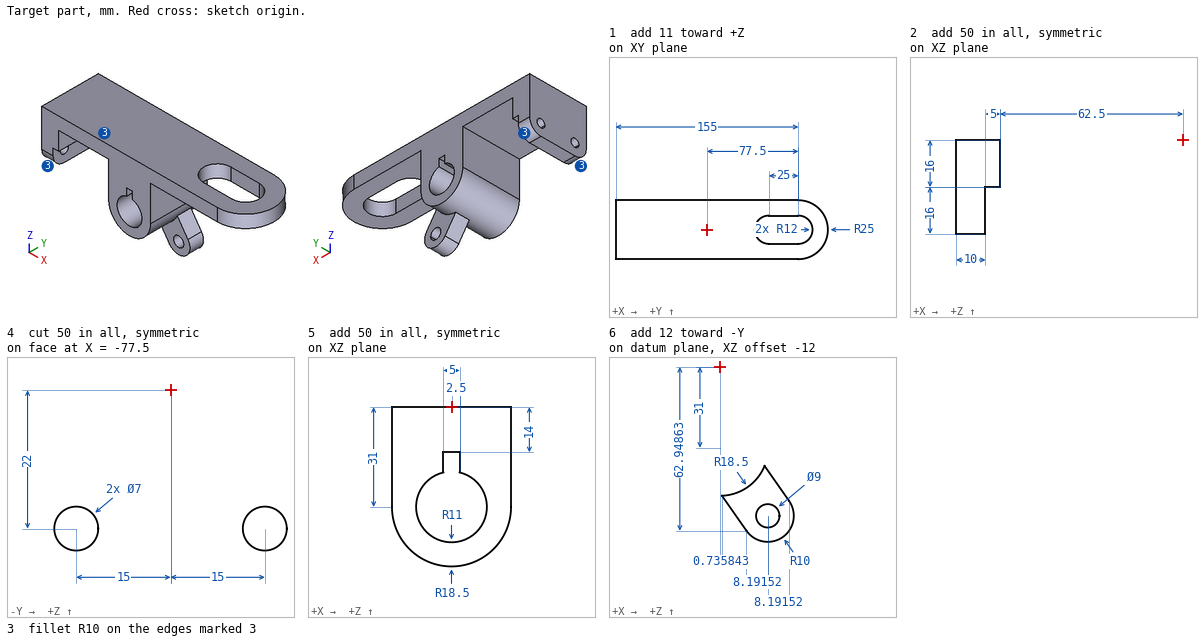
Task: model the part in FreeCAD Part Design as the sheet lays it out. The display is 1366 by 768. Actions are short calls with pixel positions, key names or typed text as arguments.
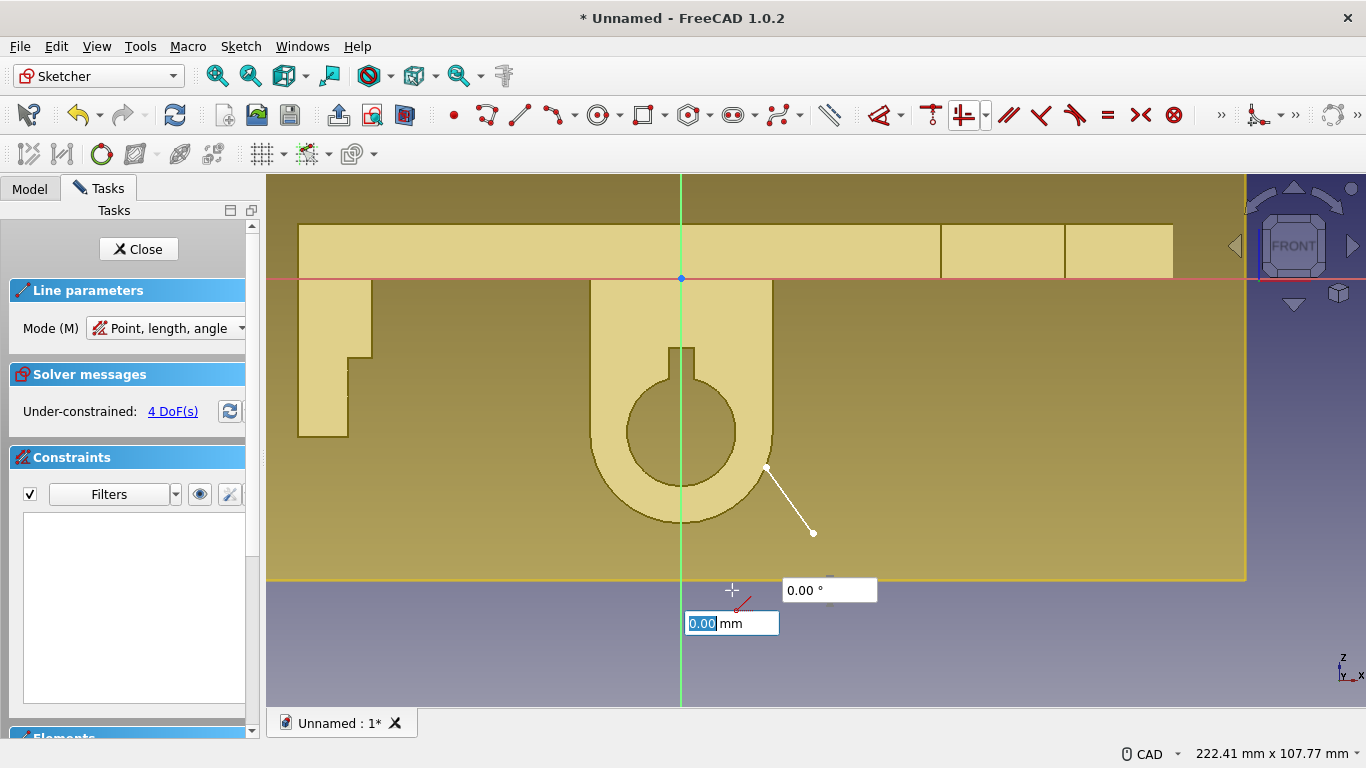
scroll(685, 523, up, 8)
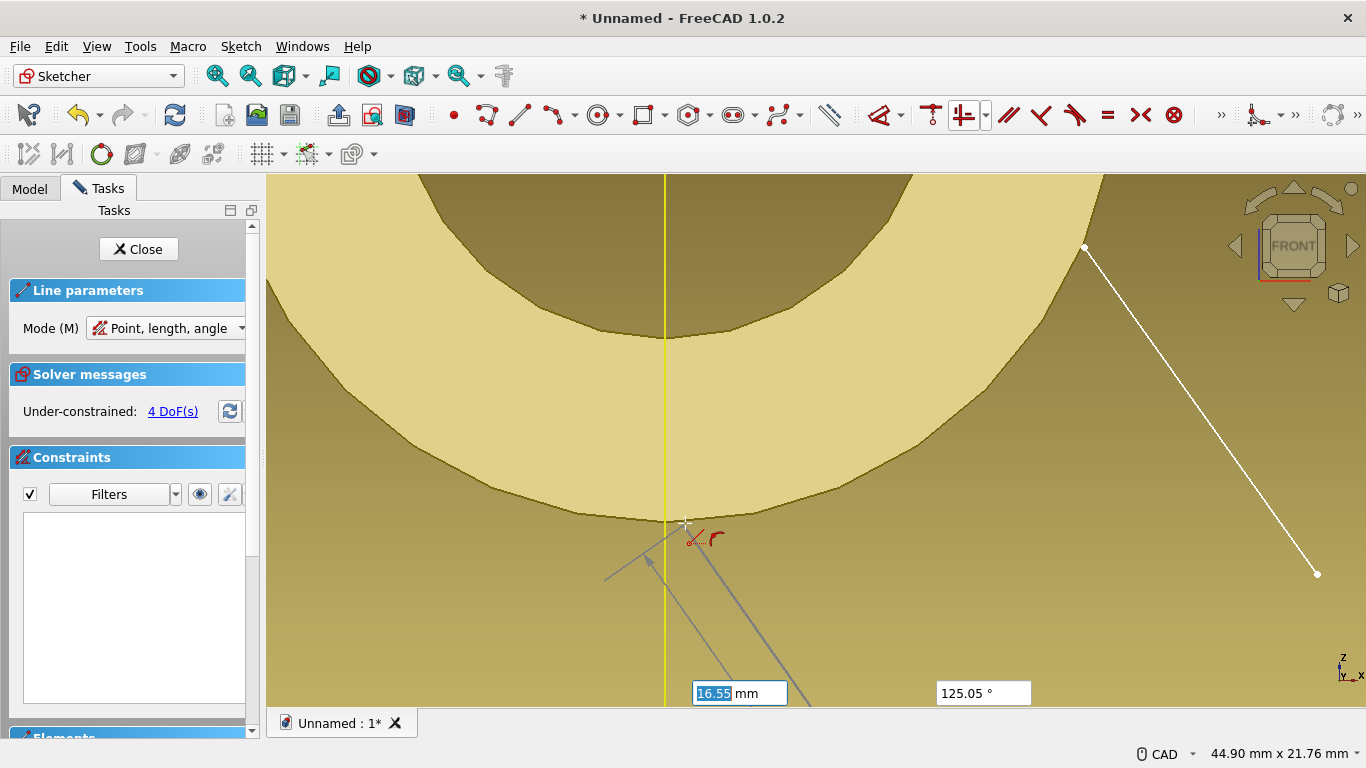
click(683, 522)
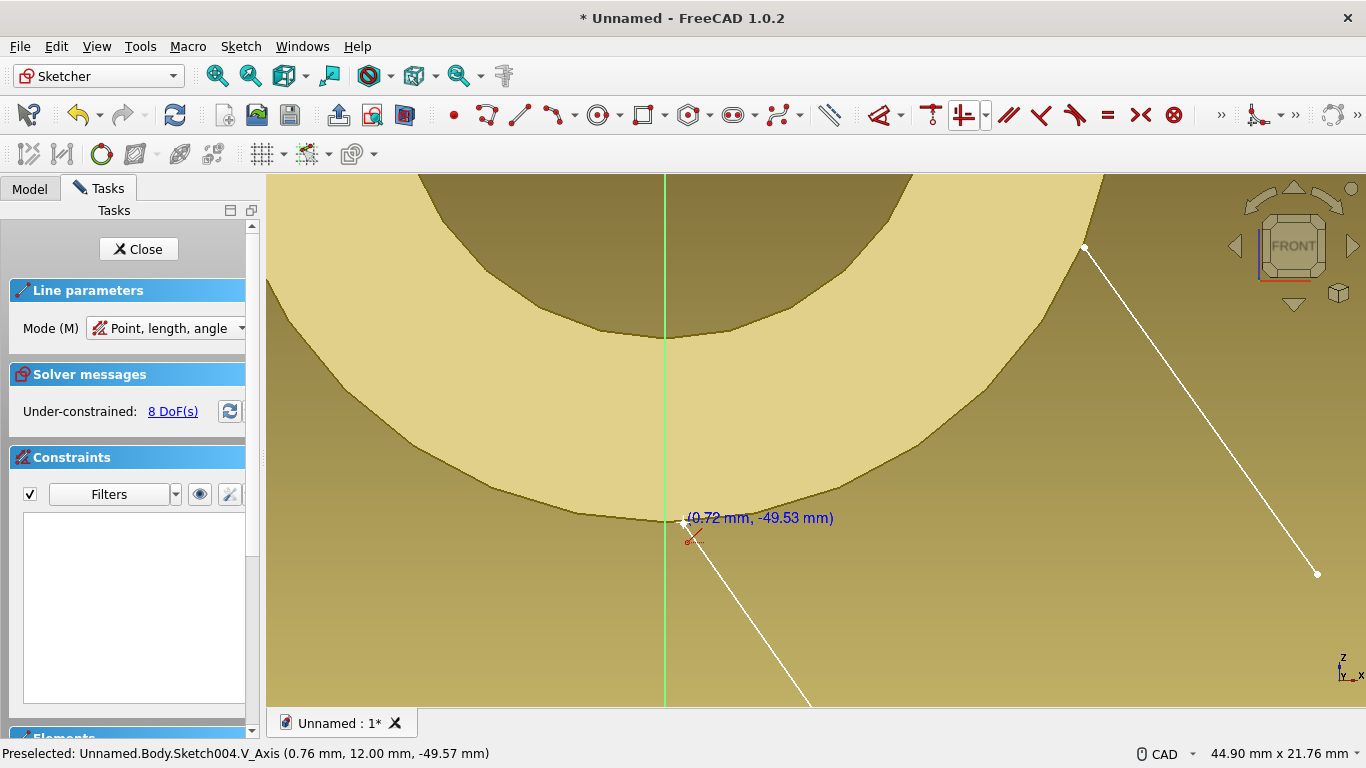
key(g)
key(3)
key(a)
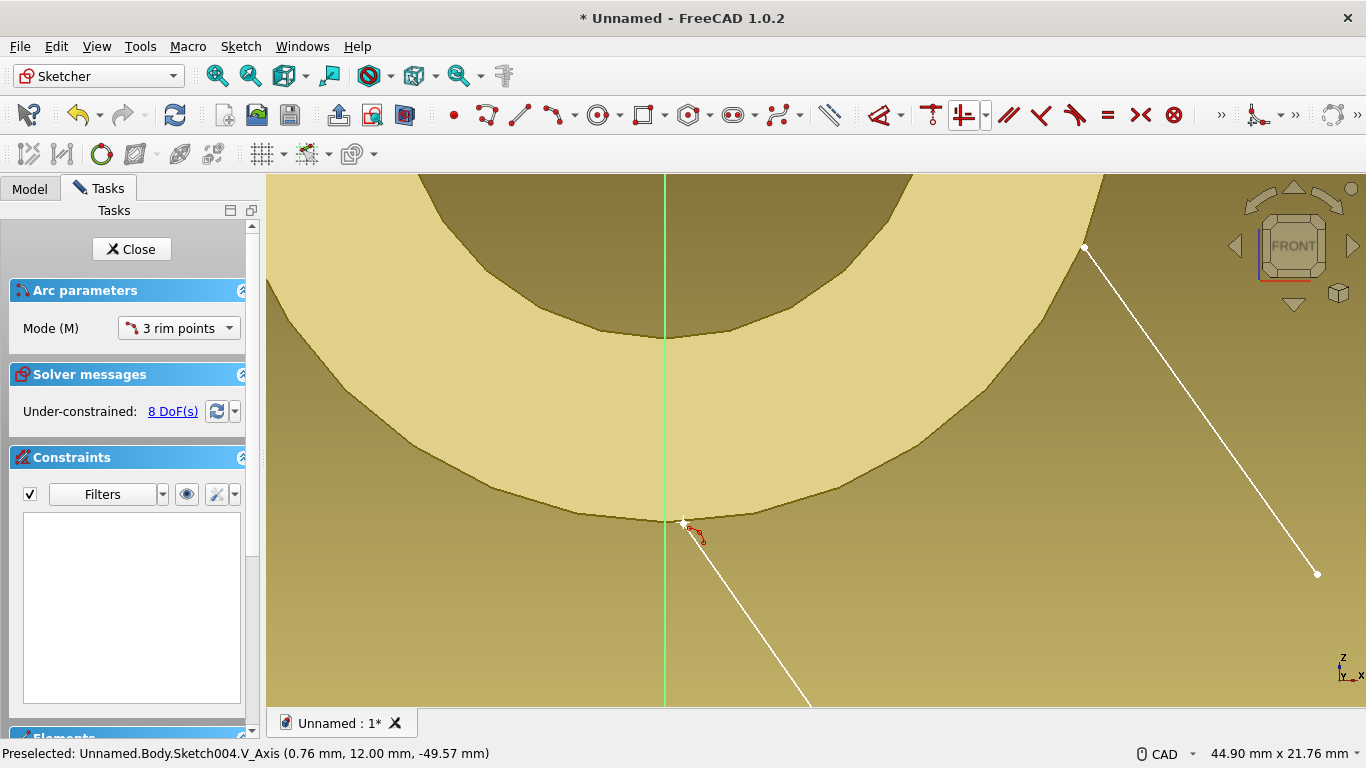
scroll(686, 524, down, 8)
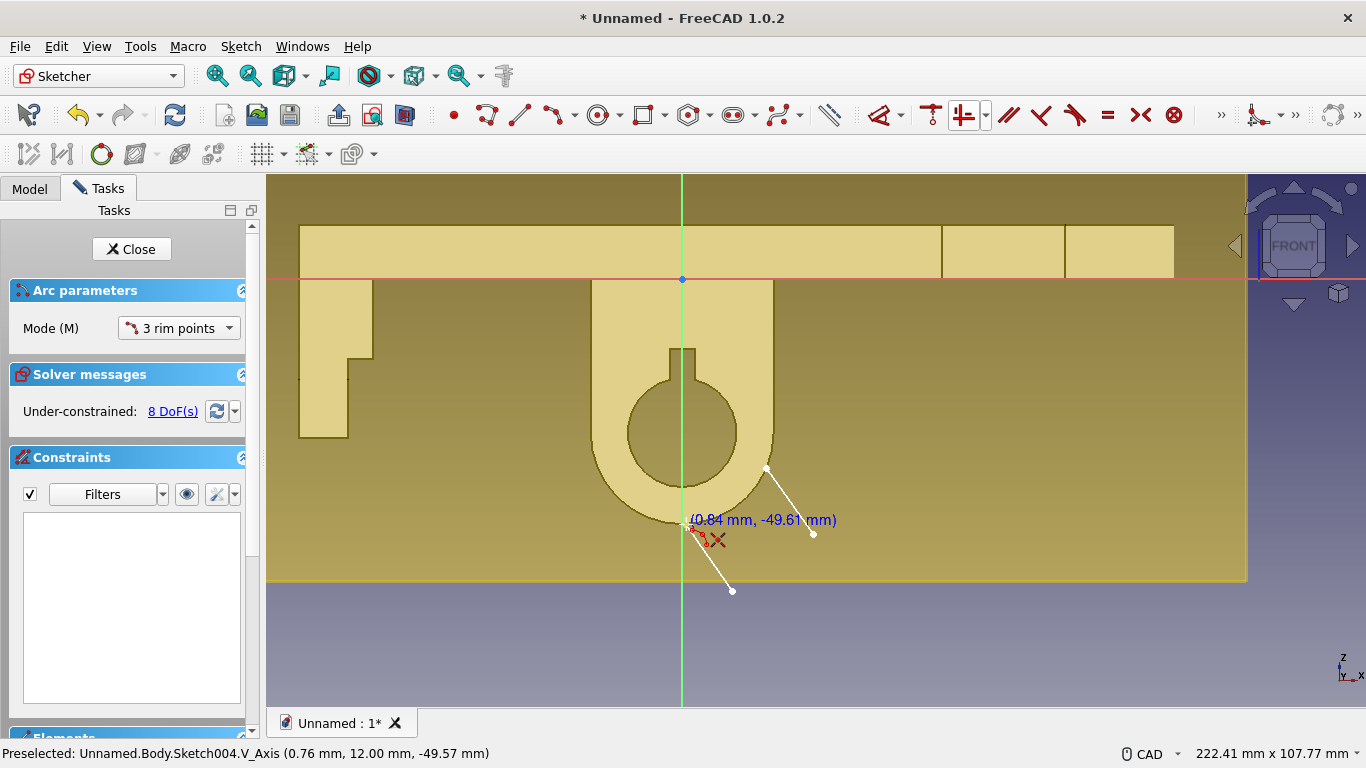
click(814, 535)
click(733, 592)
click(801, 603)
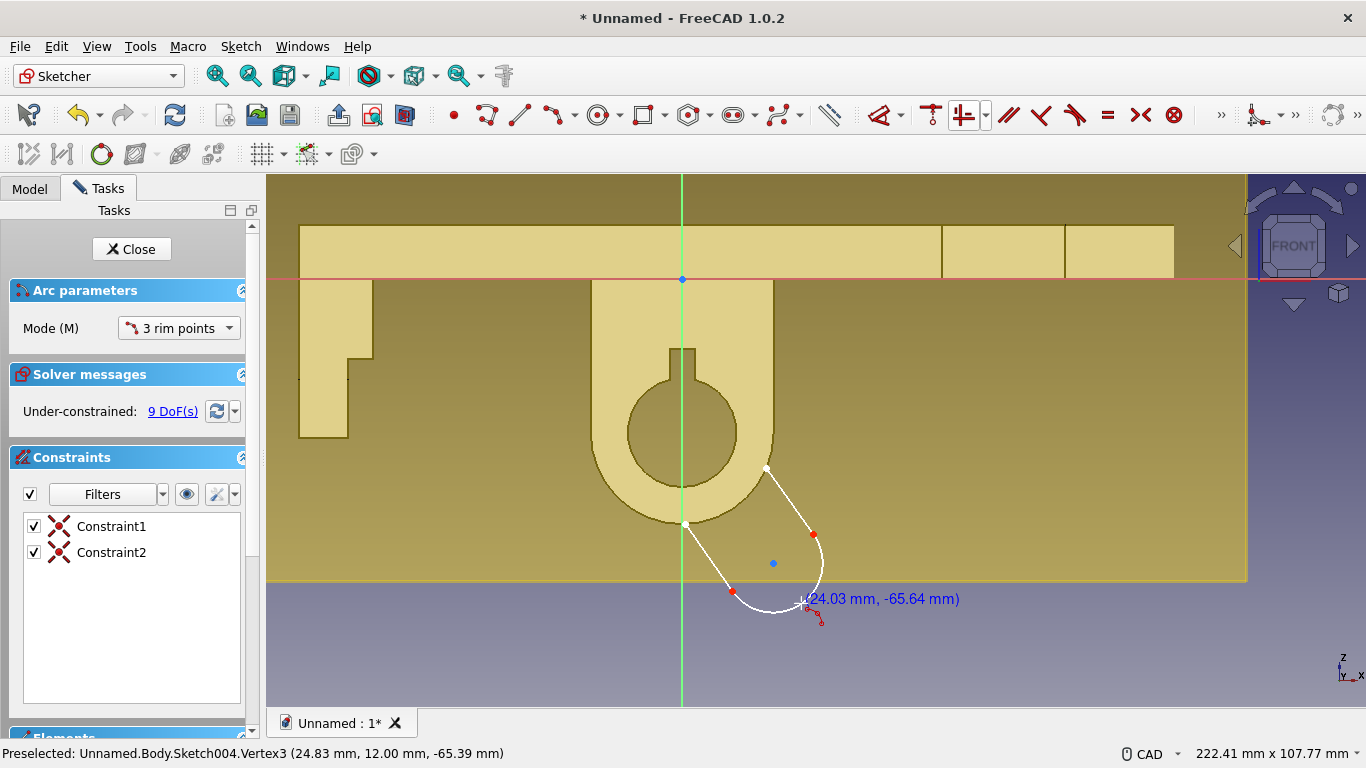
scroll(686, 524, up, 8)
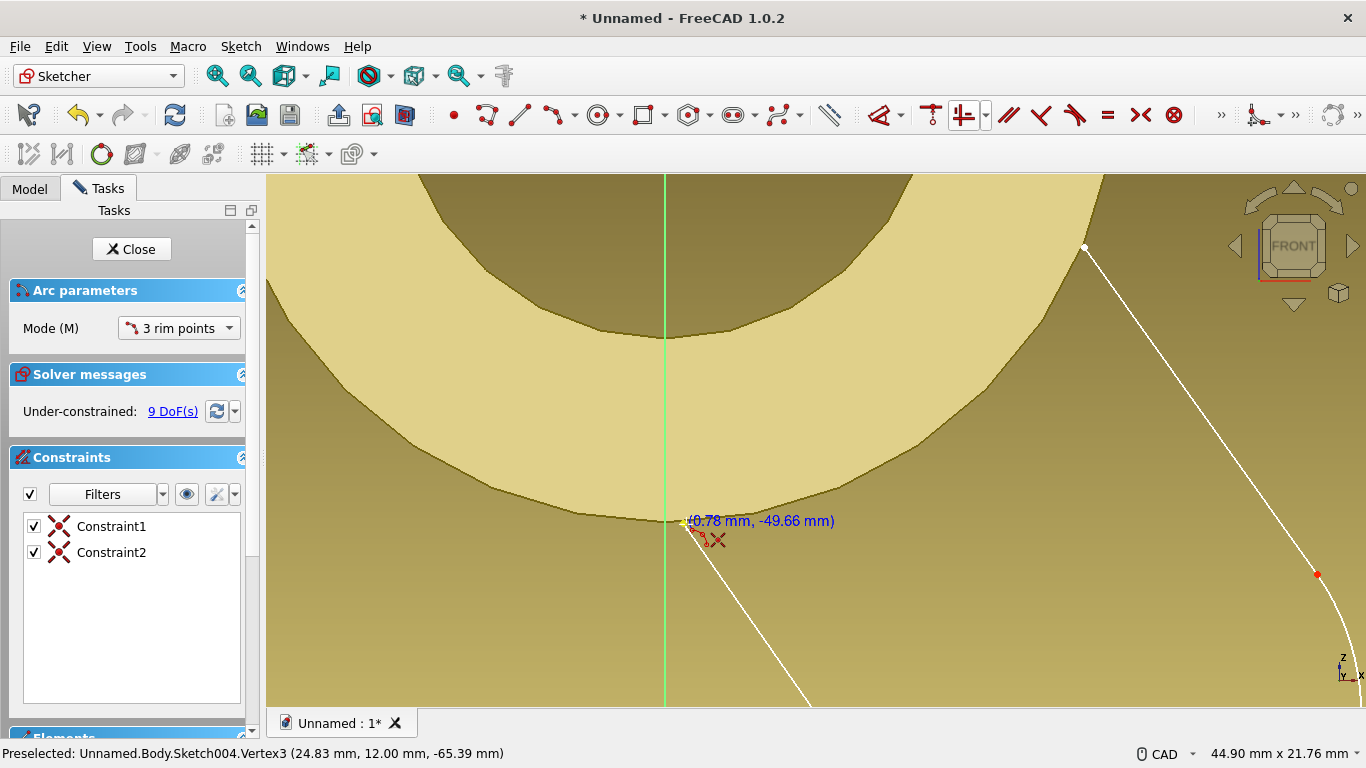
click(683, 523)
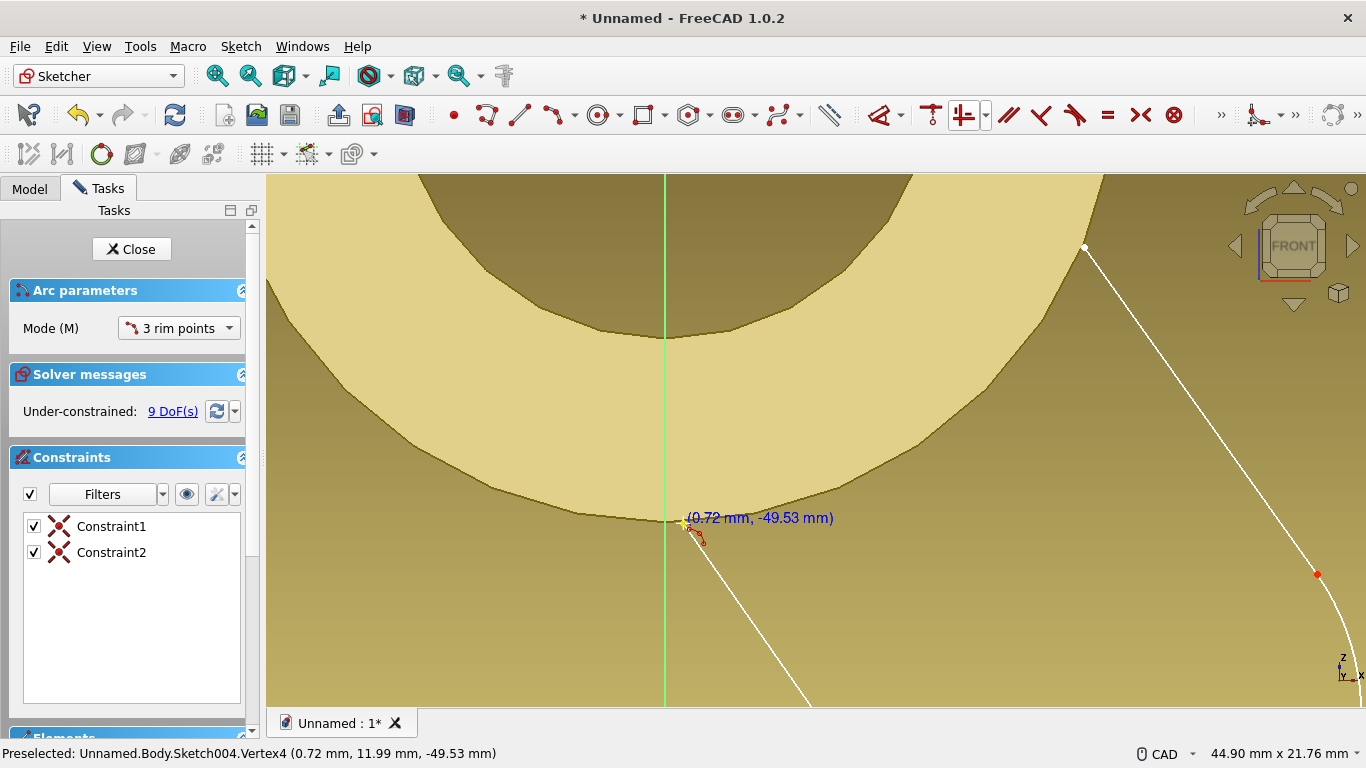
scroll(686, 524, down, 8)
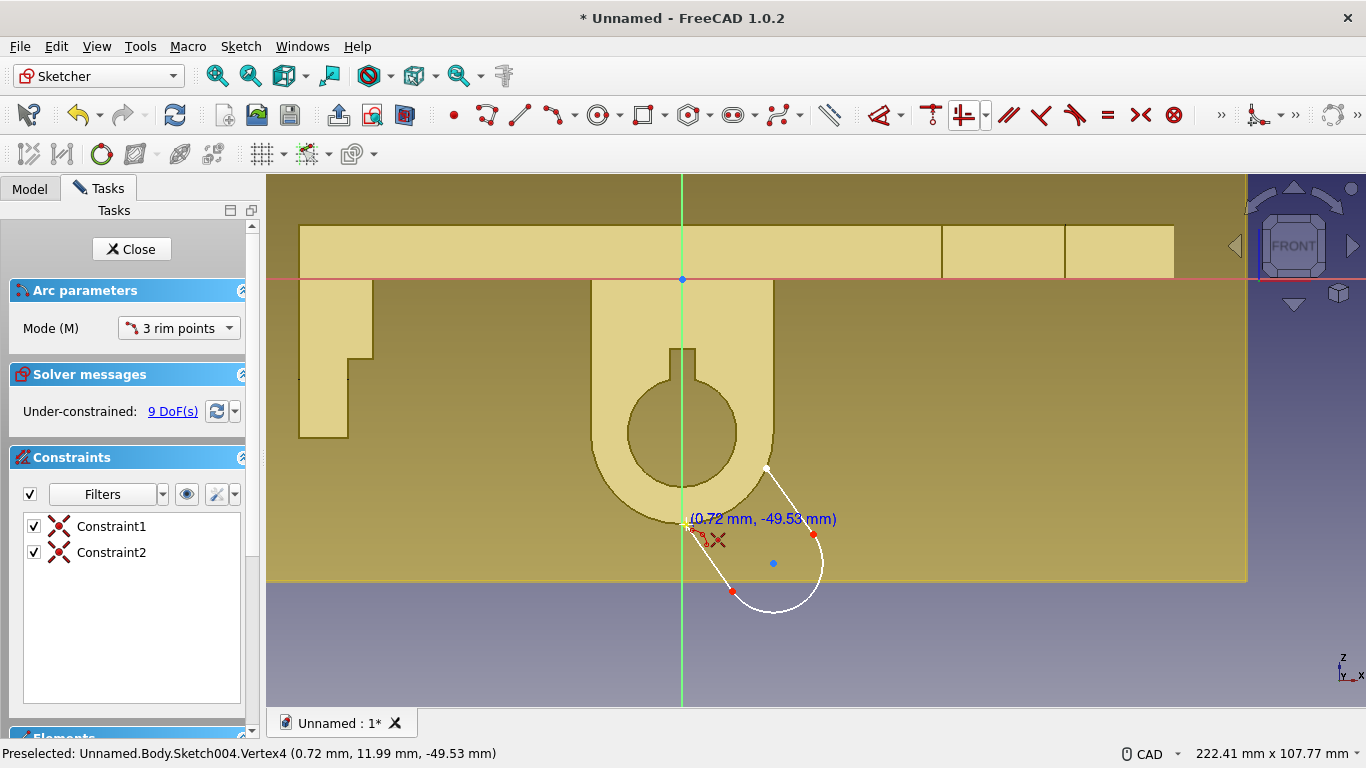
click(767, 469)
click(735, 508)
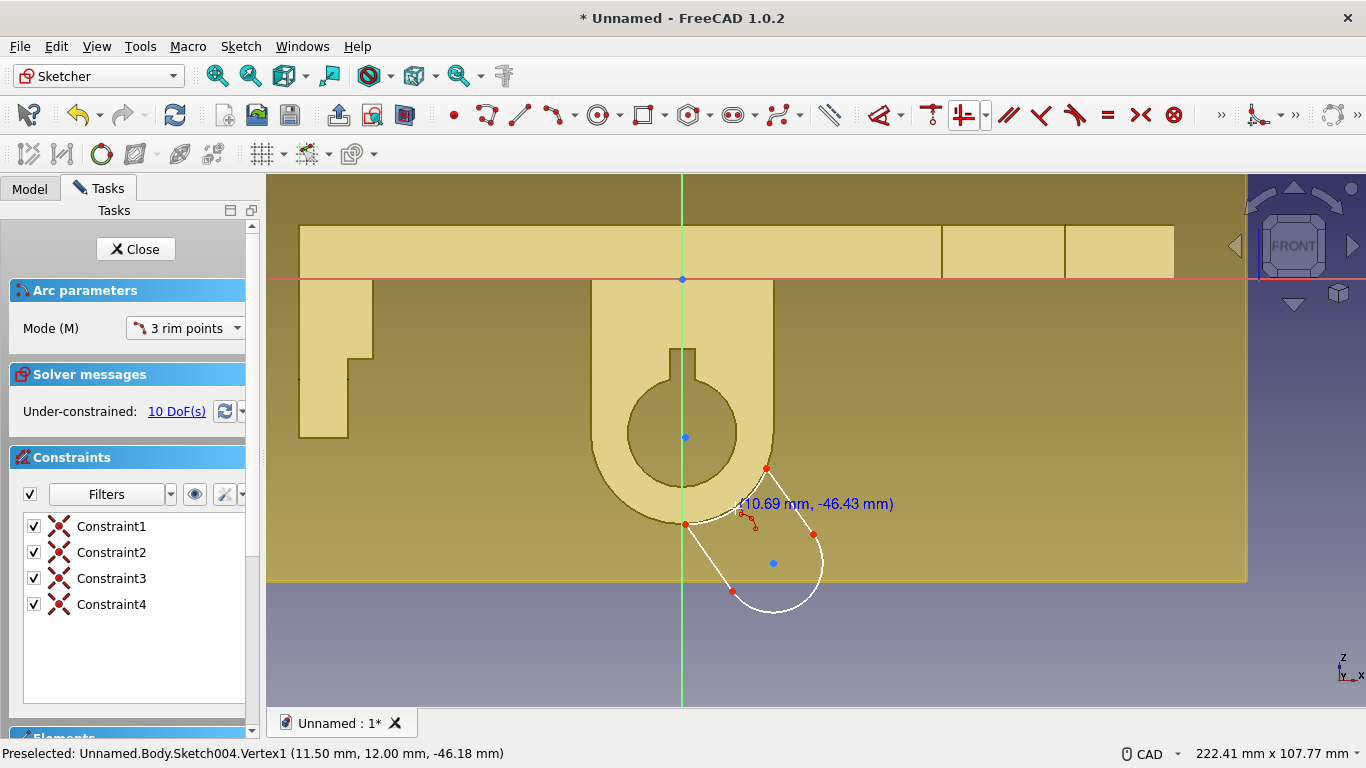
click(598, 116)